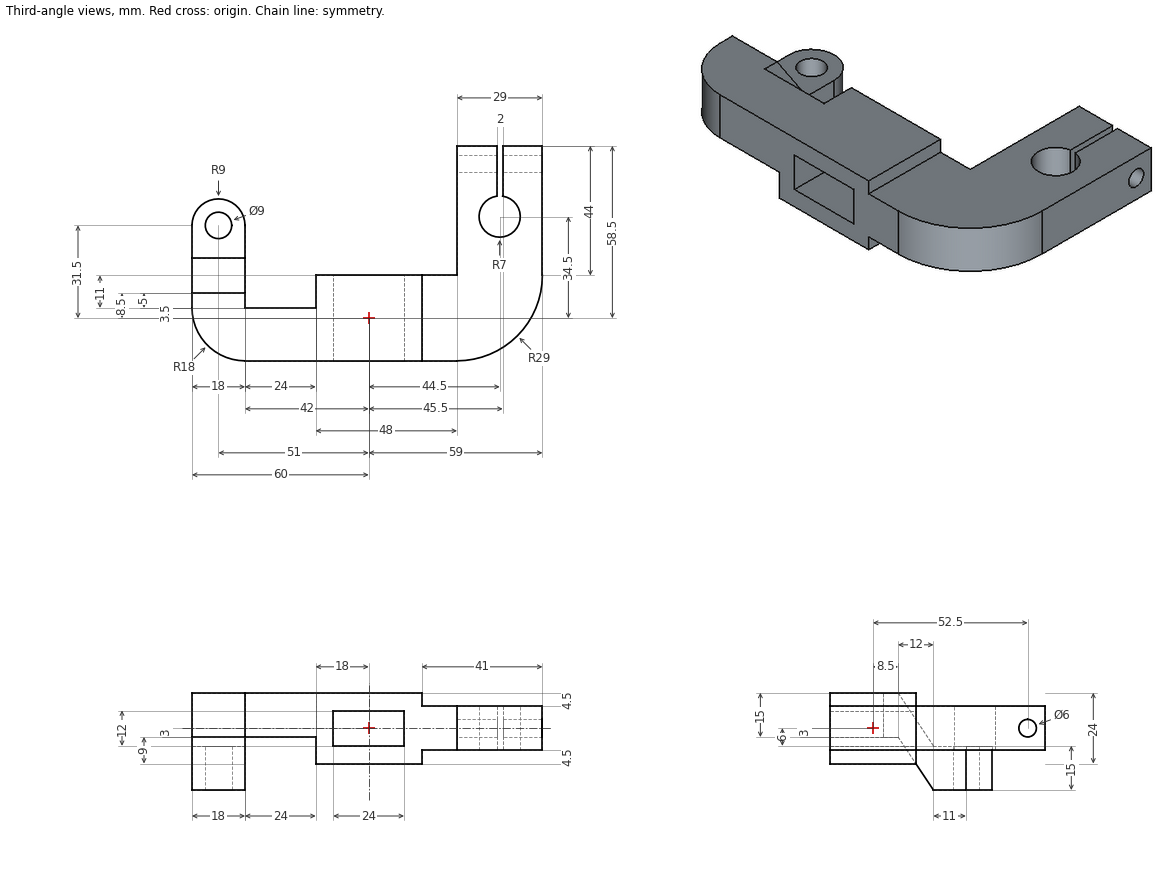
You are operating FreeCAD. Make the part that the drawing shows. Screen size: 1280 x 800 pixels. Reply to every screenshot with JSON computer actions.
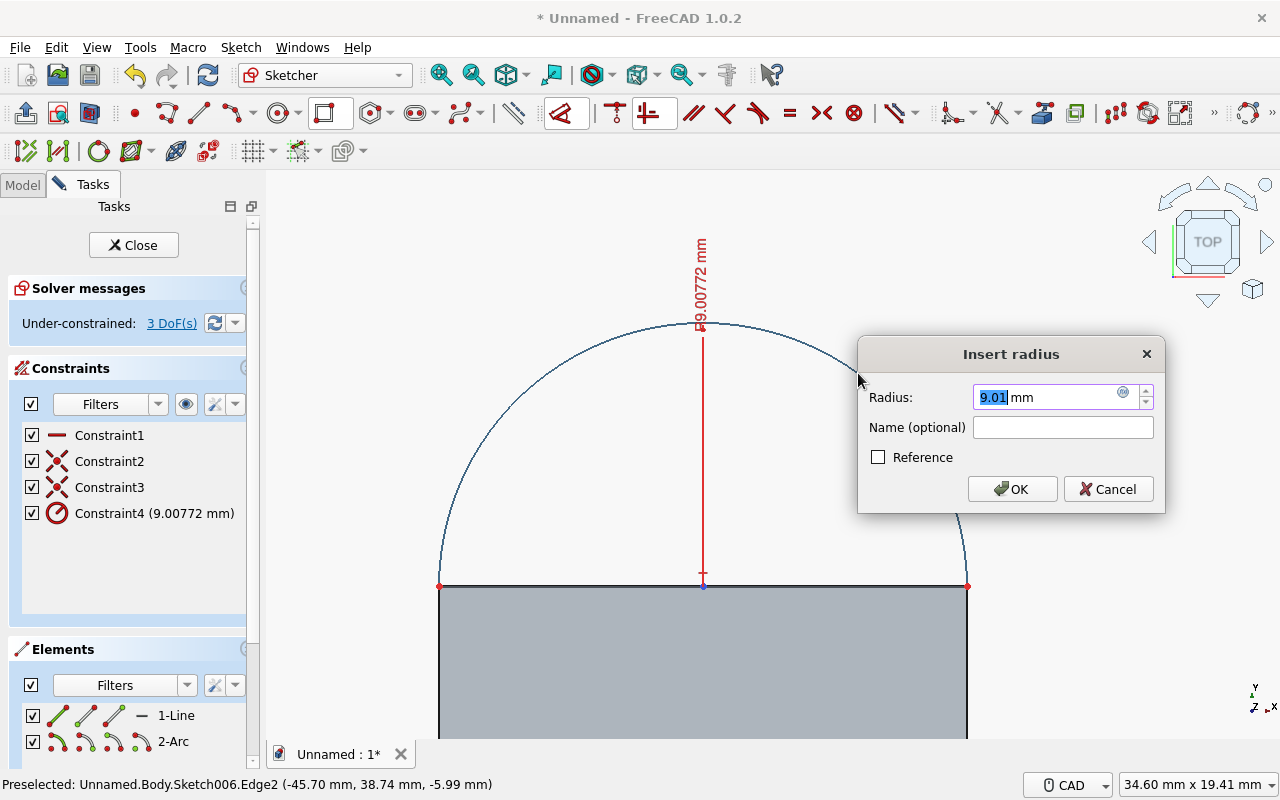
{"action": "type", "text": "9"}
{"action": "key", "text": "Return"}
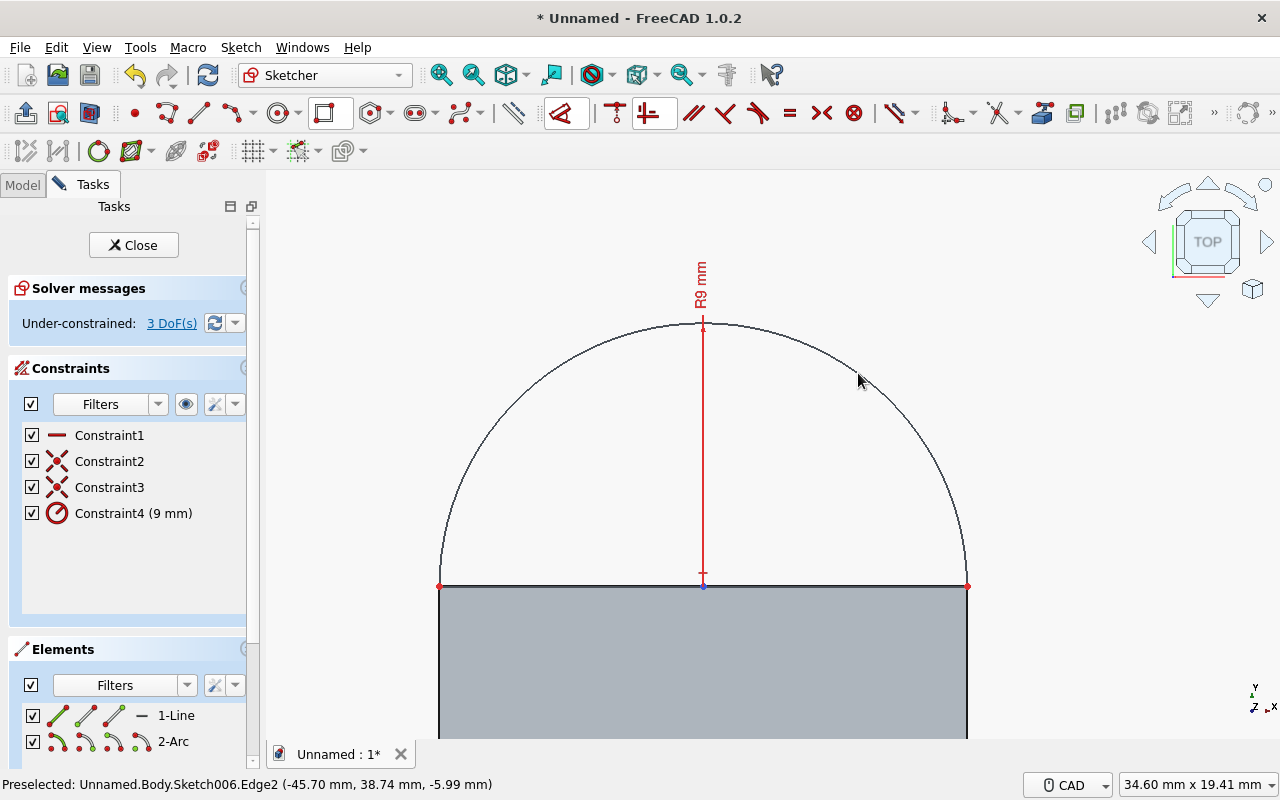
{"action": "left_click", "coordinate": [439, 587]}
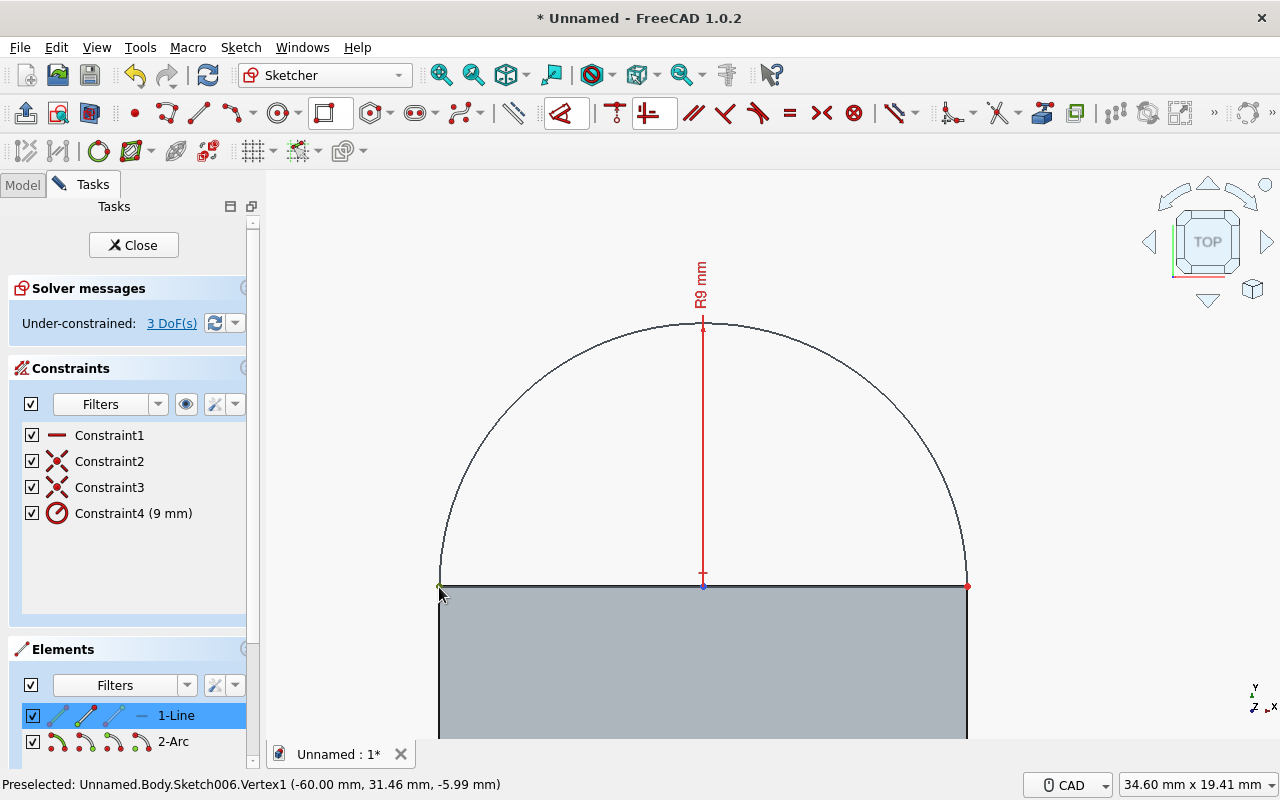
{"action": "left_click", "coordinate": [584, 114]}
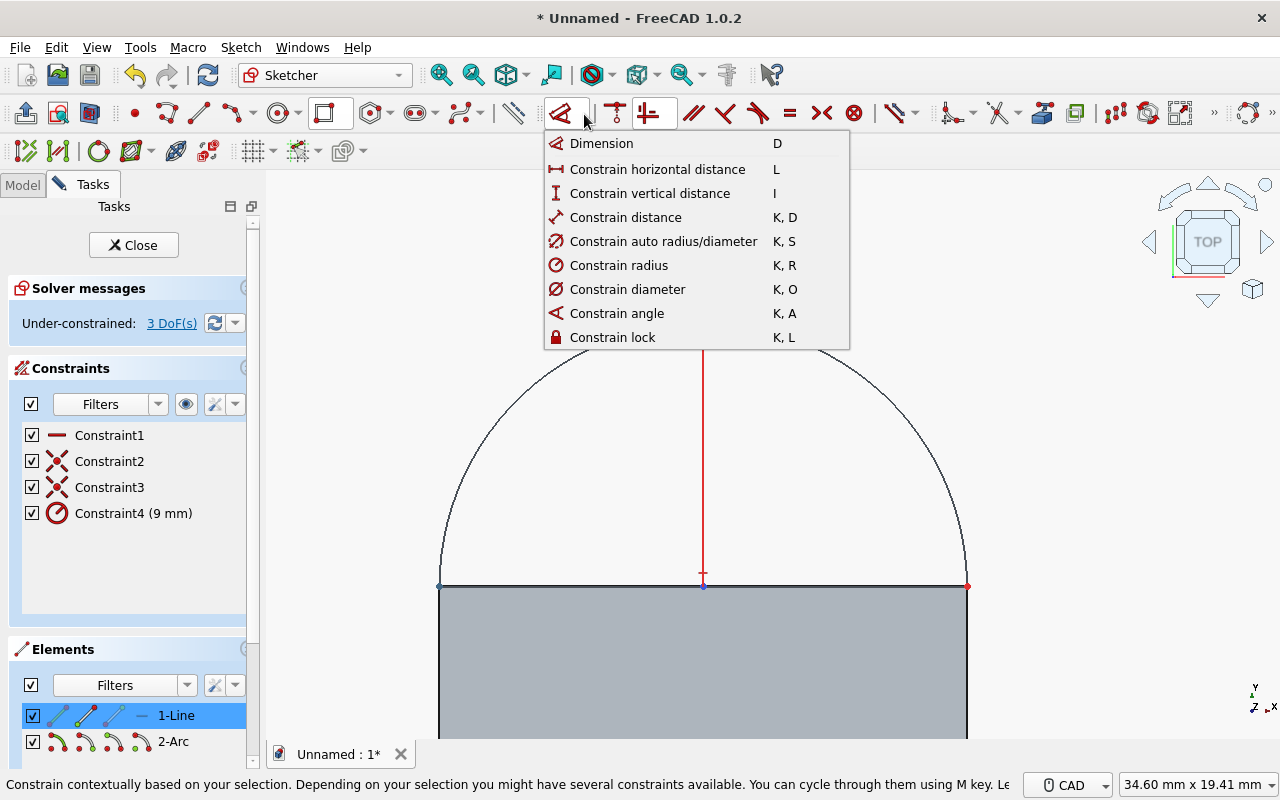
{"action": "left_click", "coordinate": [697, 169]}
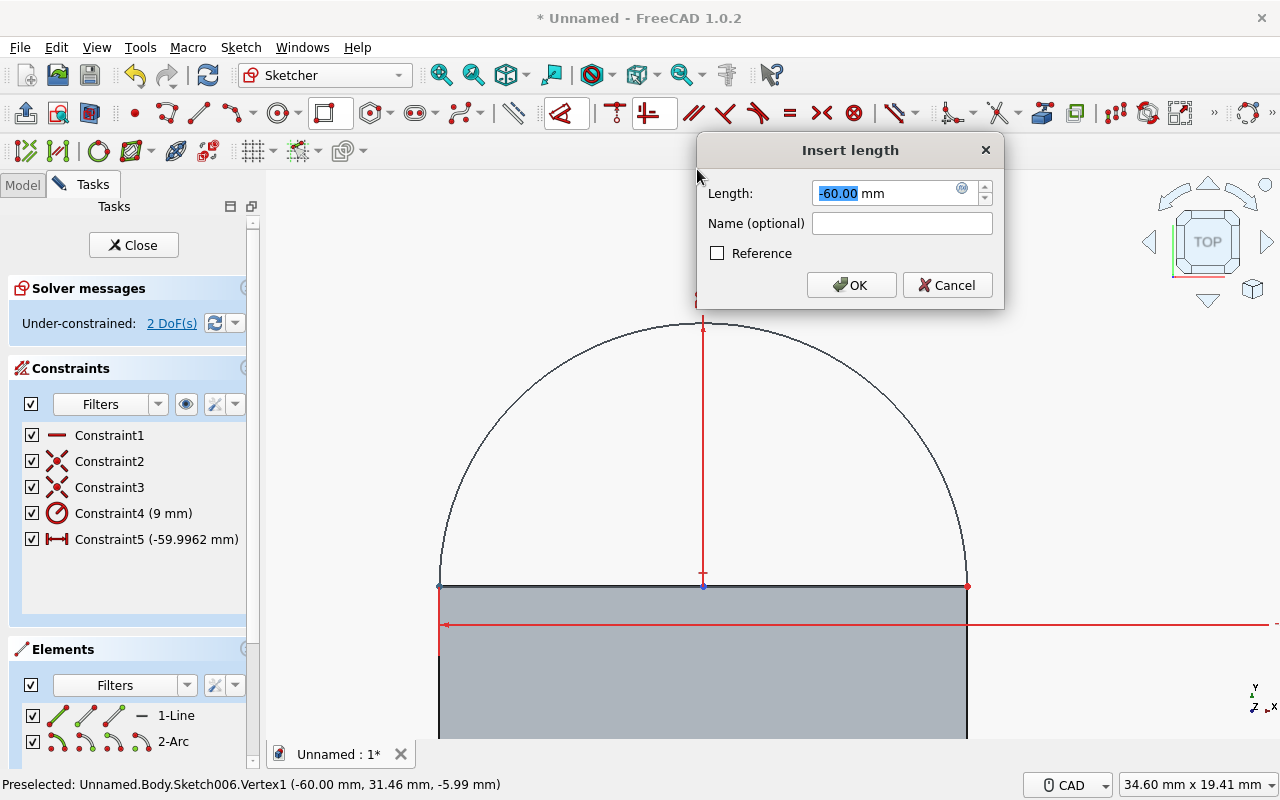
{"action": "type", "text": "-60"}
{"action": "key", "text": "Return"}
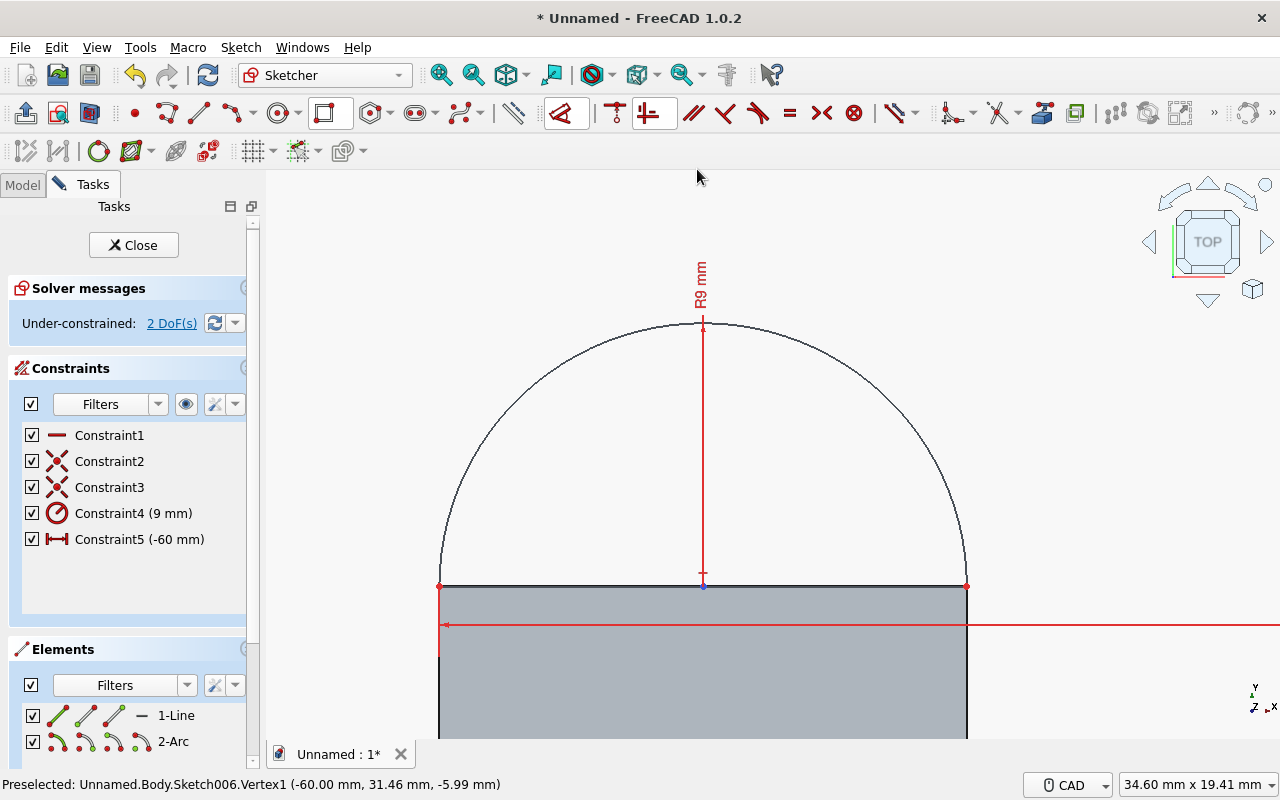
{"action": "left_click", "coordinate": [439, 587]}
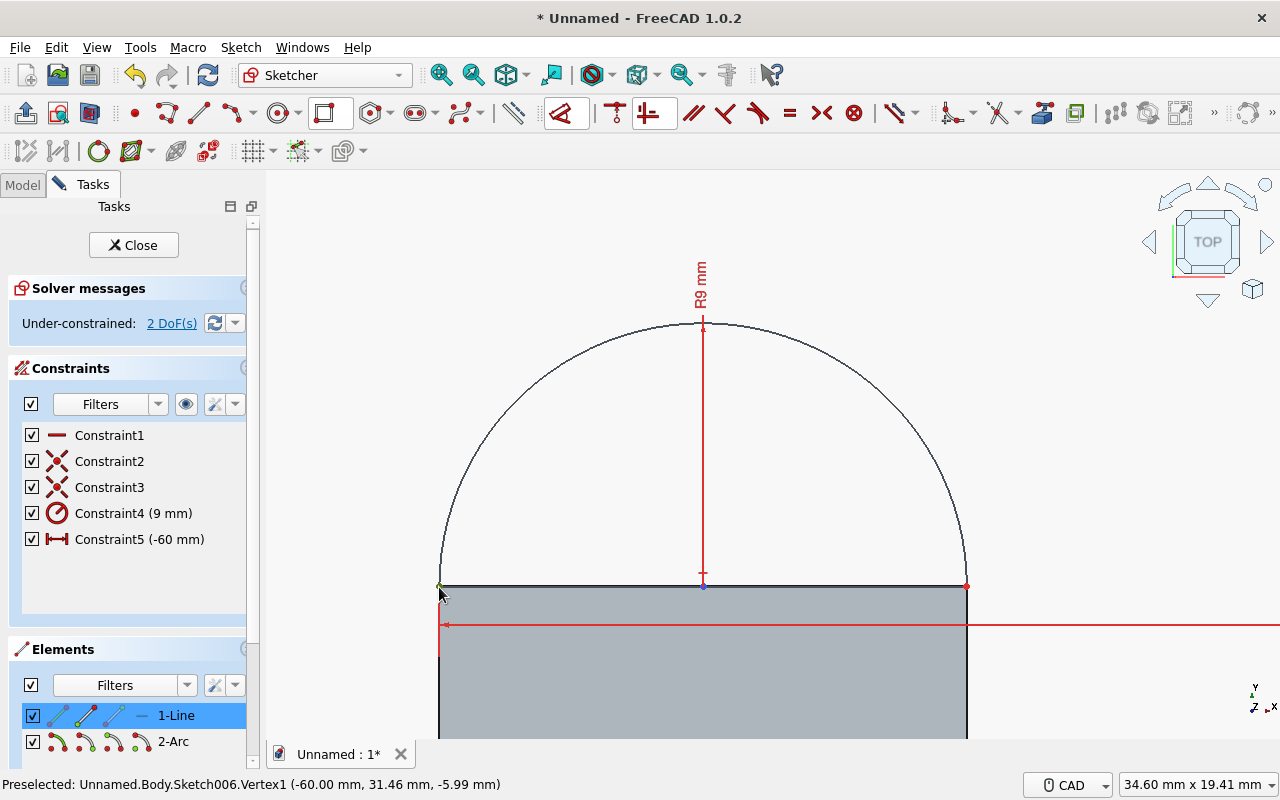
{"action": "left_click", "coordinate": [584, 114]}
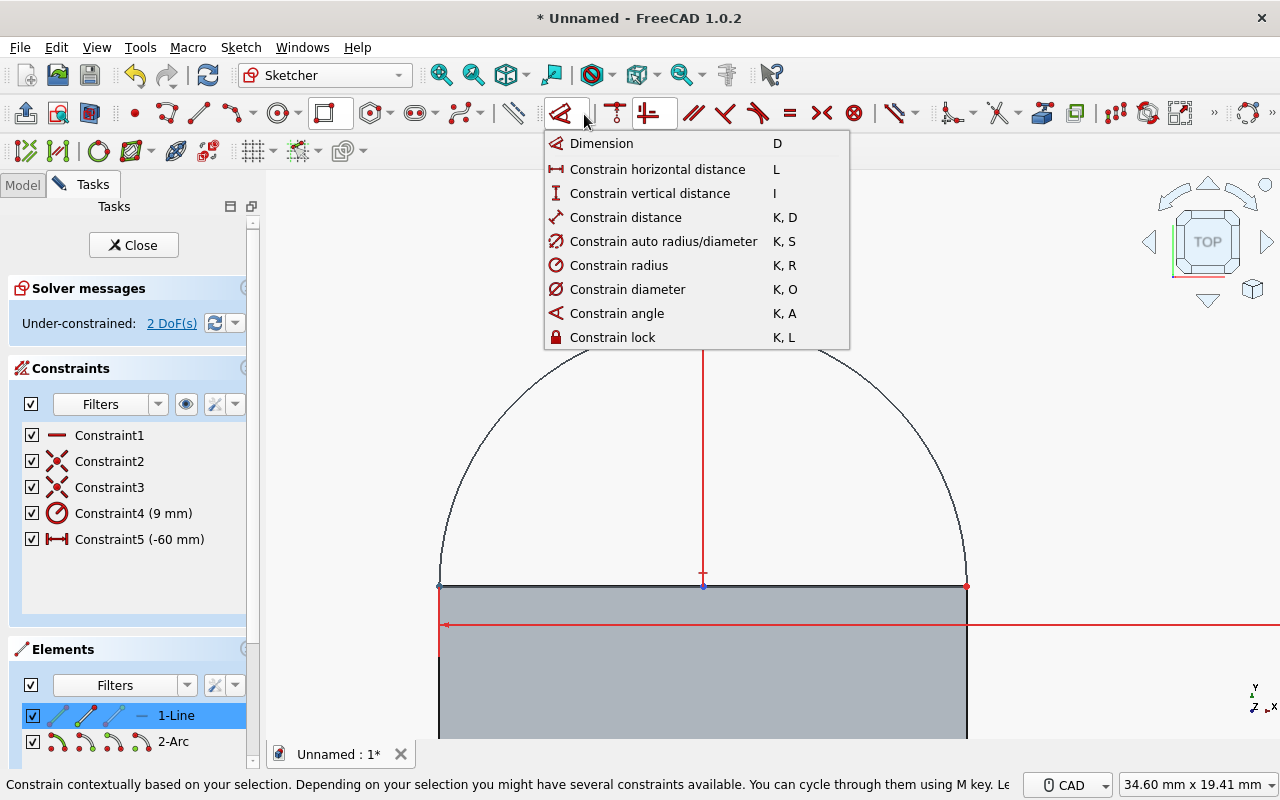
{"action": "left_click", "coordinate": [697, 193]}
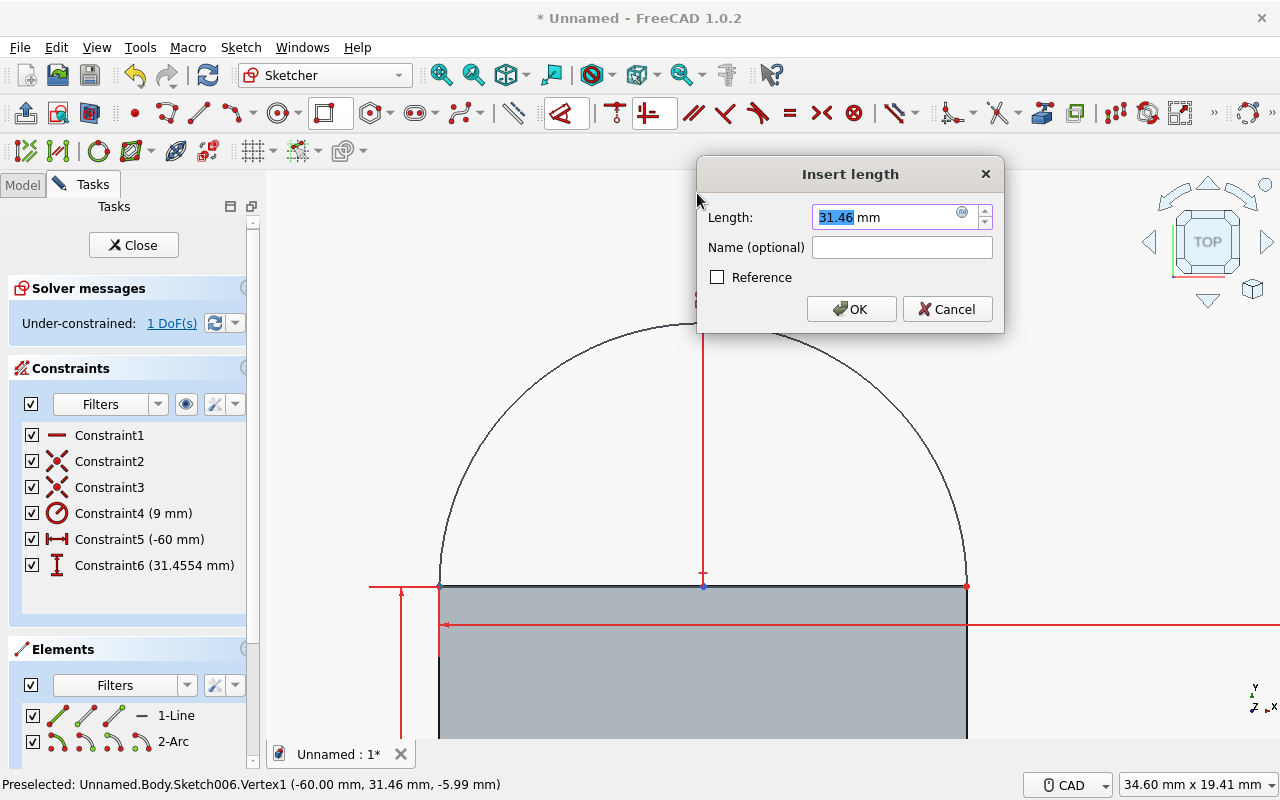
{"action": "type", "text": "31.5"}
{"action": "key", "text": "Return"}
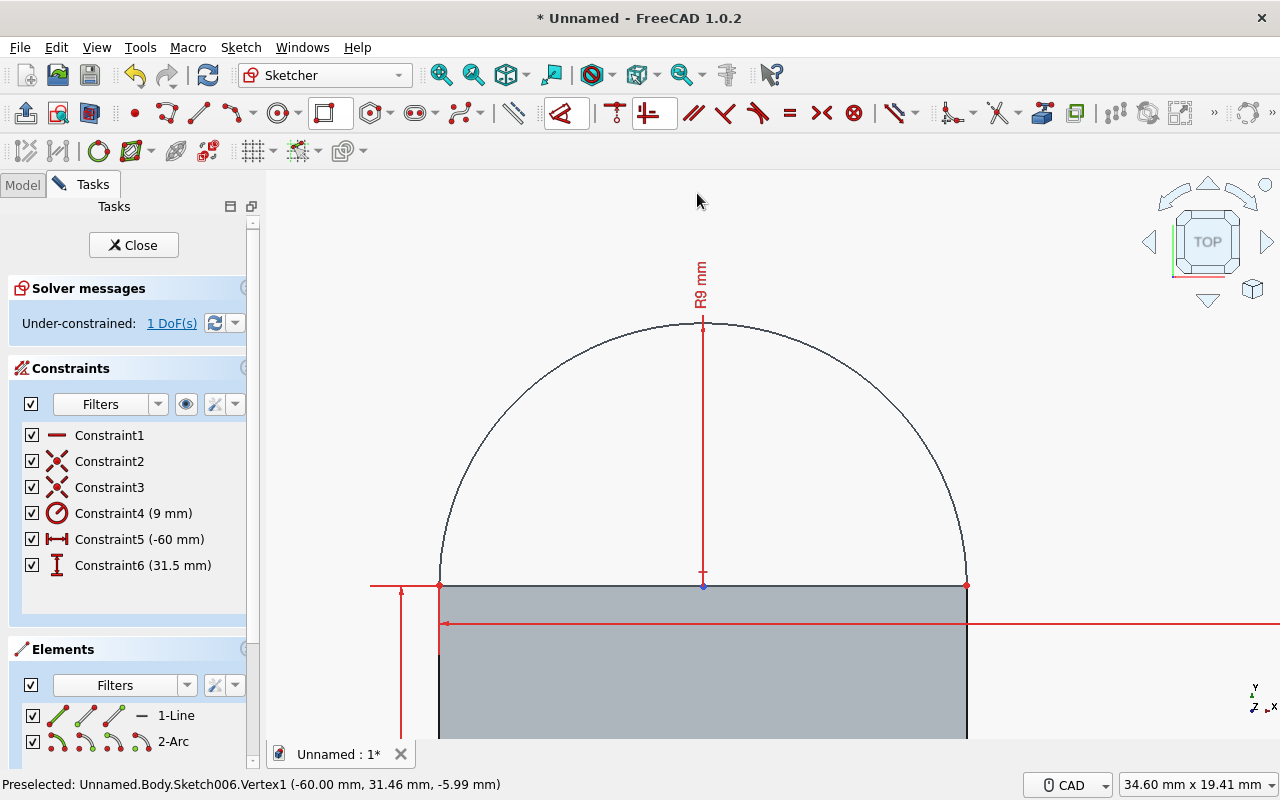
{"action": "left_click", "coordinate": [703, 587]}